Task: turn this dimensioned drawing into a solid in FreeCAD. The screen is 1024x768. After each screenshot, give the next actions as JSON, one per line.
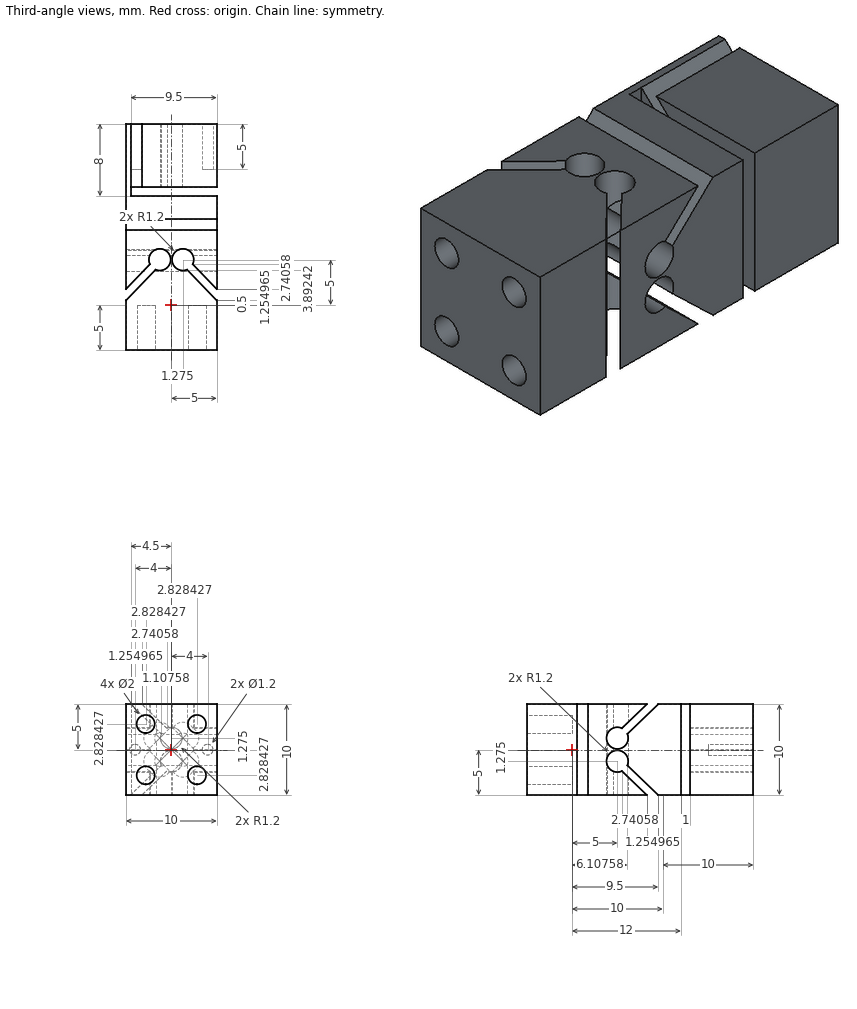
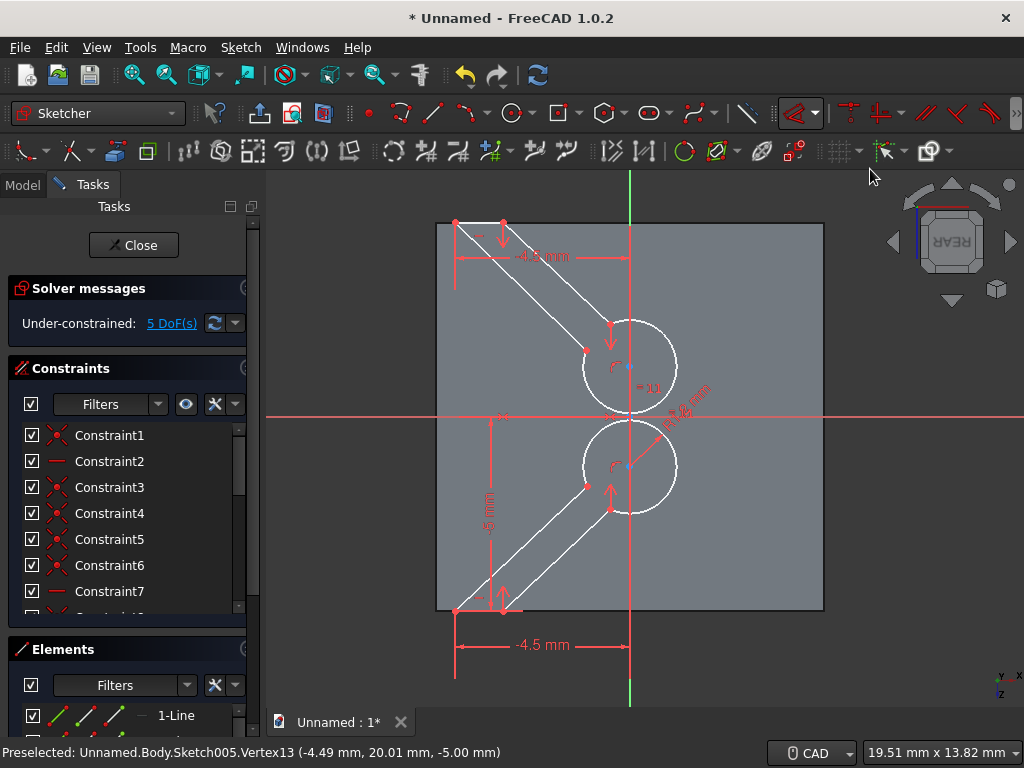
{"action": "left_click", "coordinate": [630, 467]}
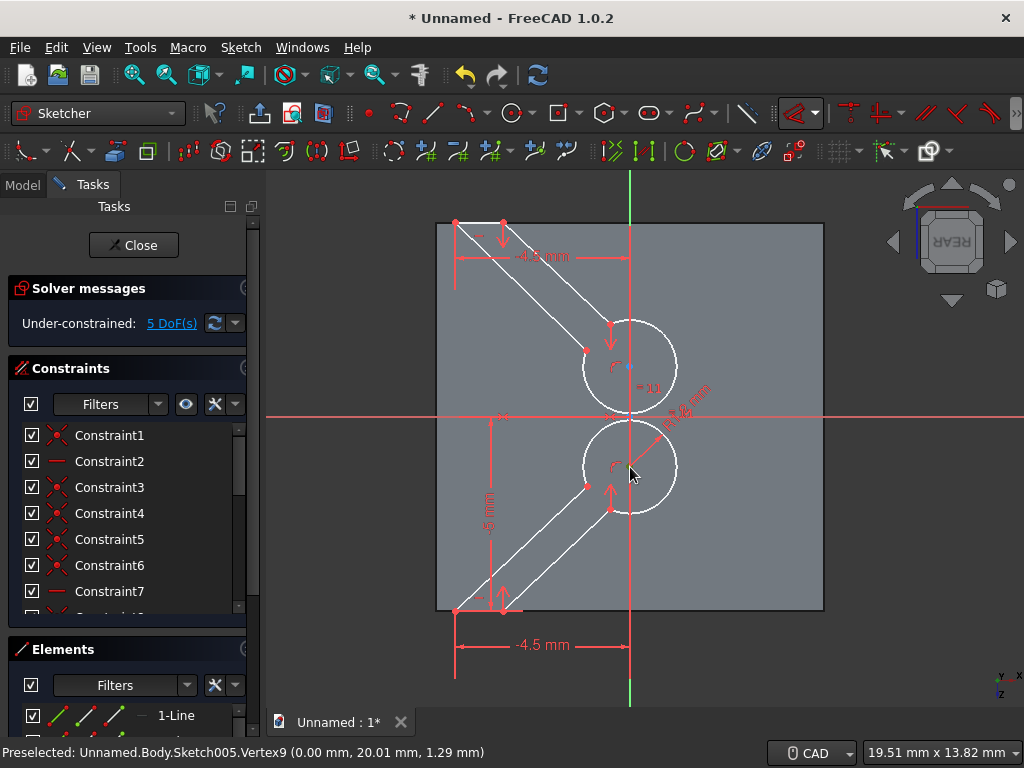
{"action": "key", "text": "i"}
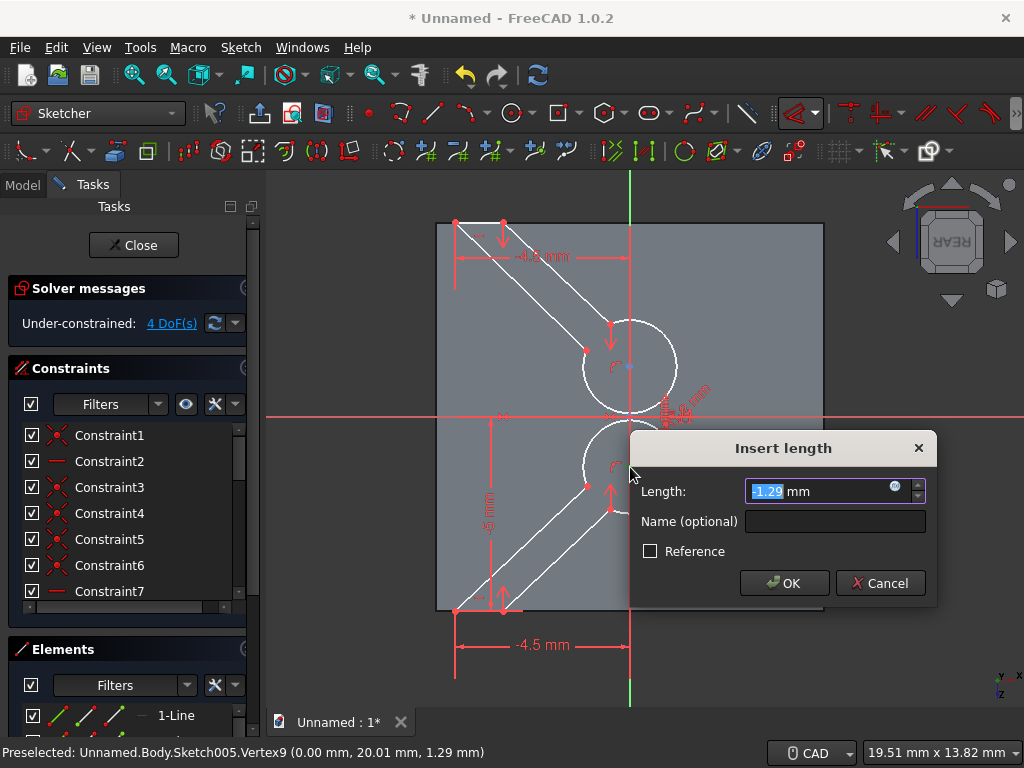
{"action": "type", "text": "-1.275"}
{"action": "key", "text": "Return"}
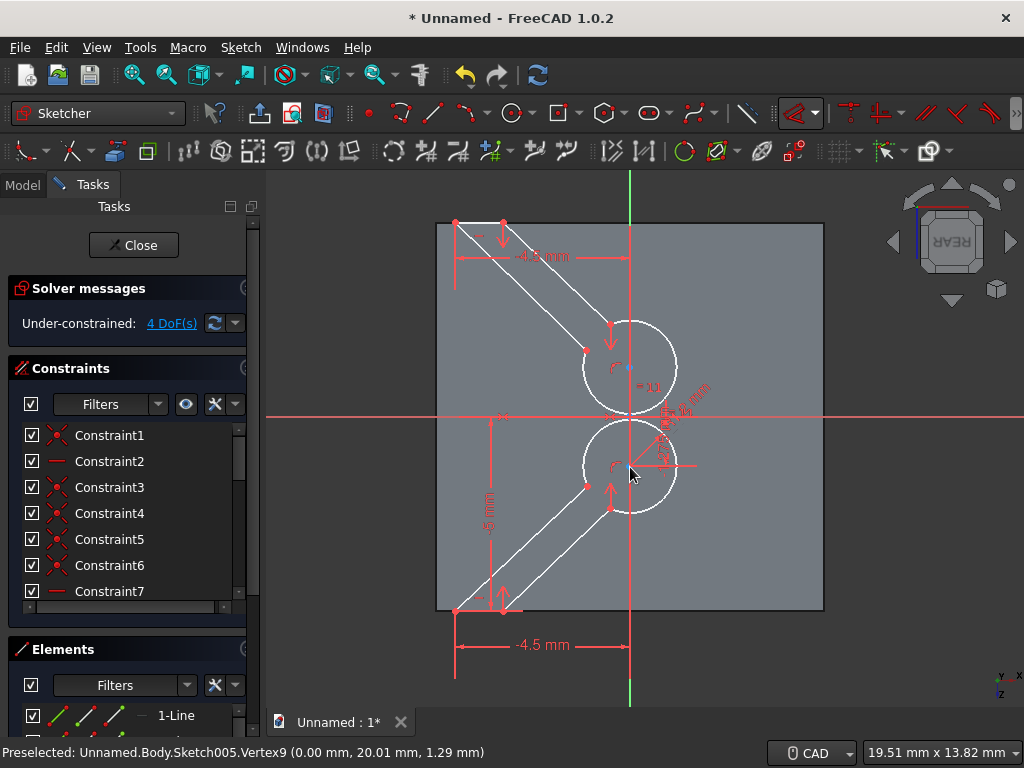
{"action": "scroll", "coordinate": [470, 611], "scroll_direction": "up", "scroll_amount": 2}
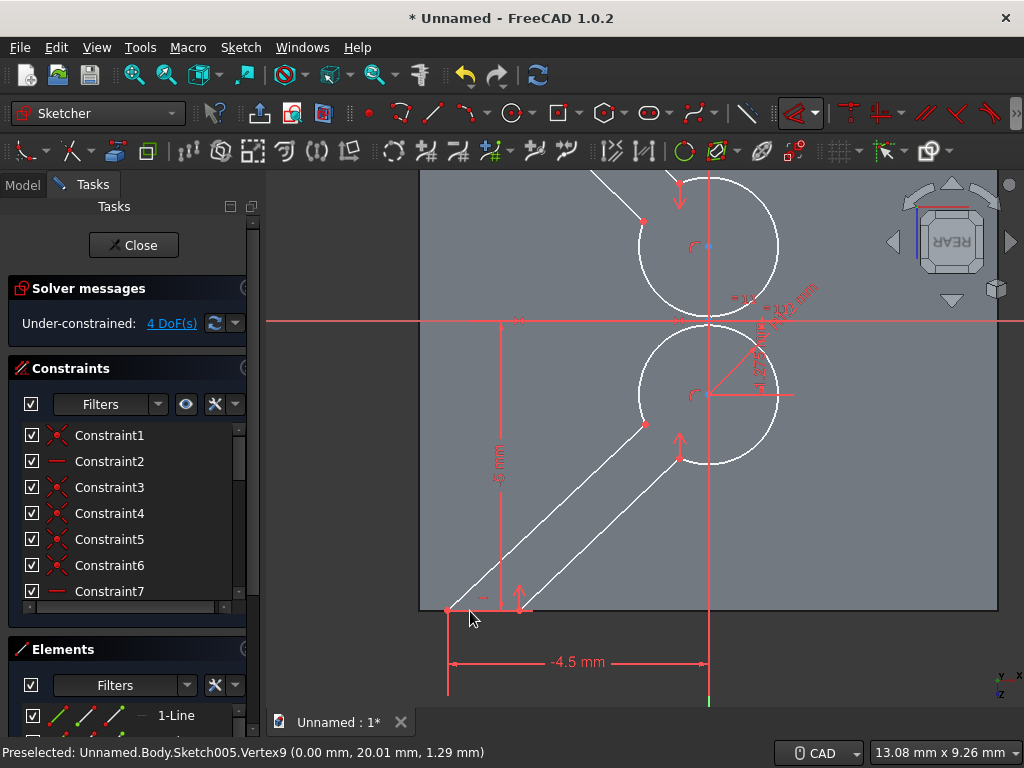
{"action": "left_click", "coordinate": [469, 611]}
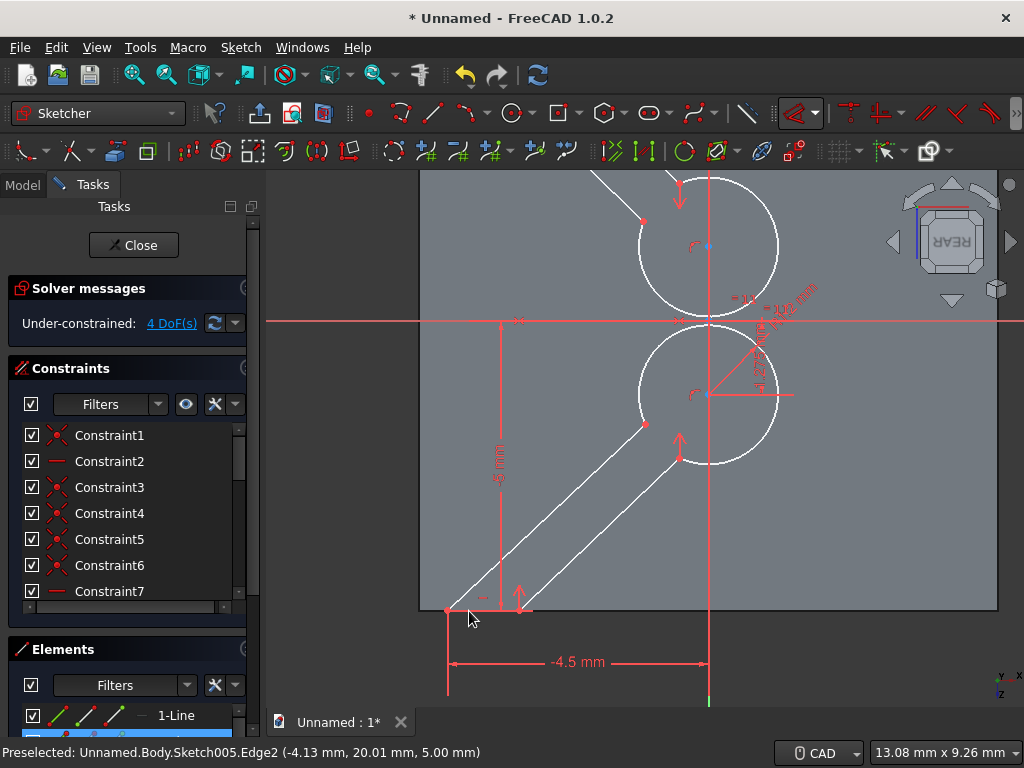
{"action": "key", "text": "l"}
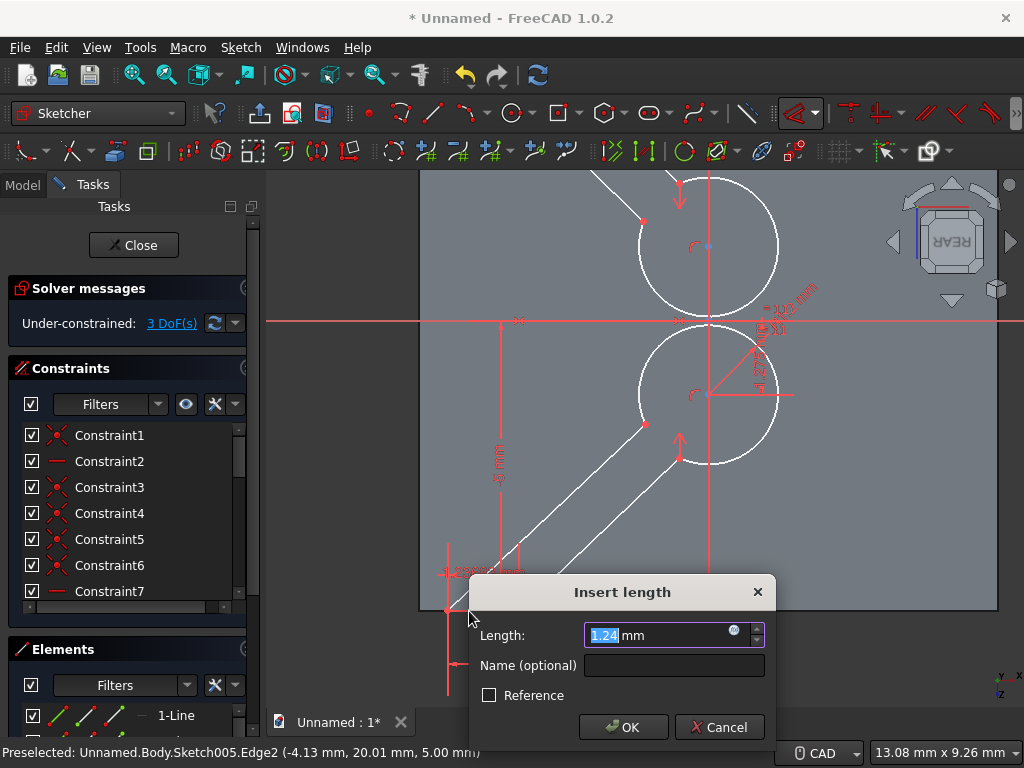
{"action": "type", "text": "1.254965"}
{"action": "key", "text": "Return"}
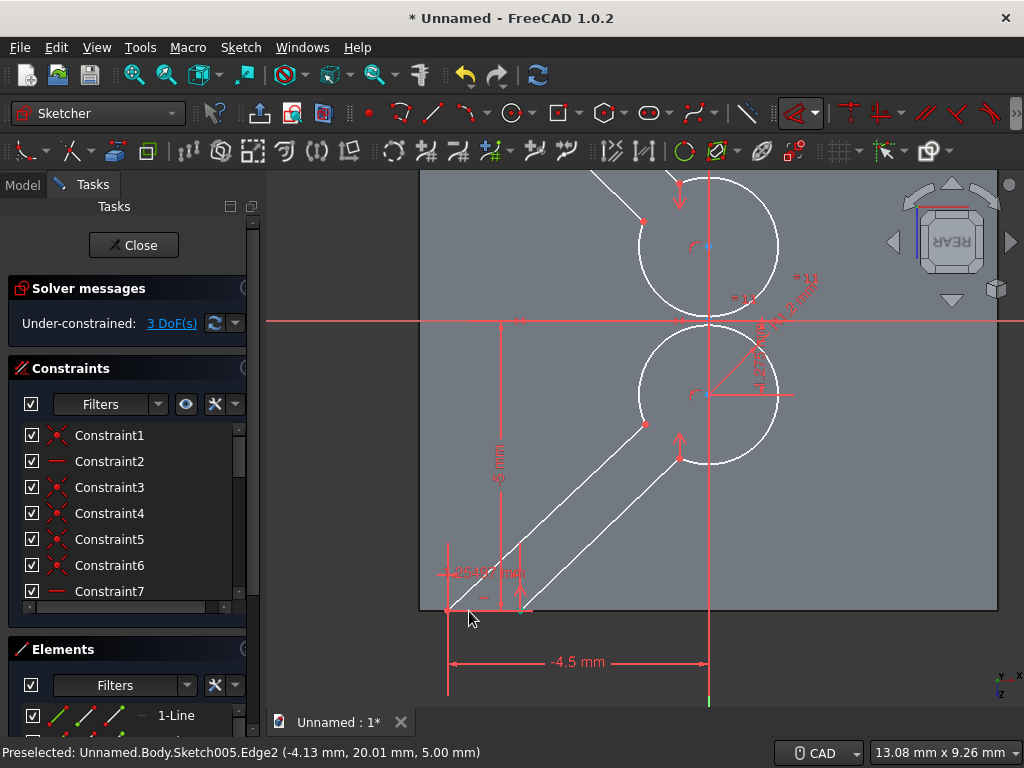
{"action": "left_click", "coordinate": [646, 424]}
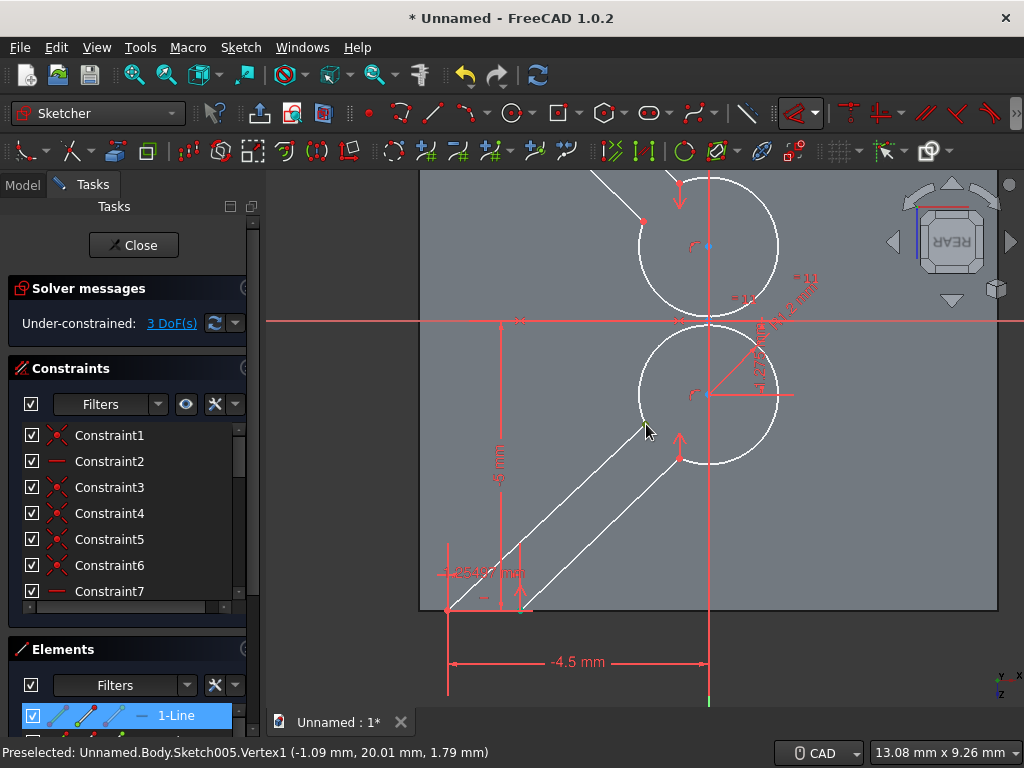
{"action": "key", "text": "l"}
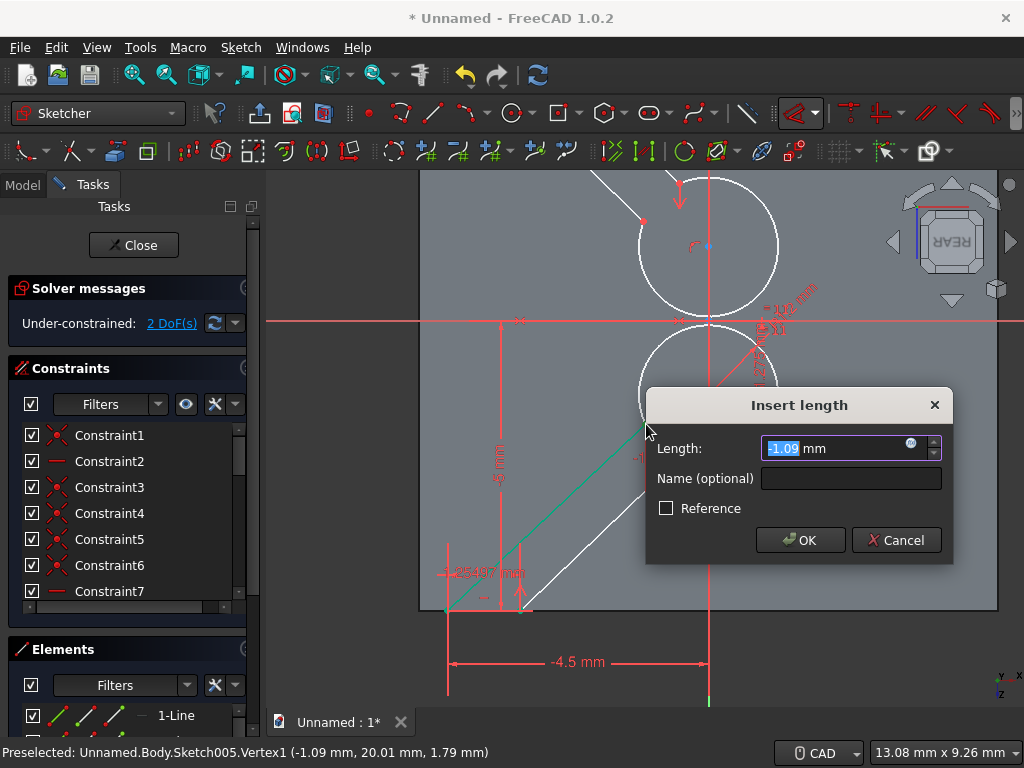
{"action": "type", "text": "-1.10758"}
{"action": "key", "text": "Return"}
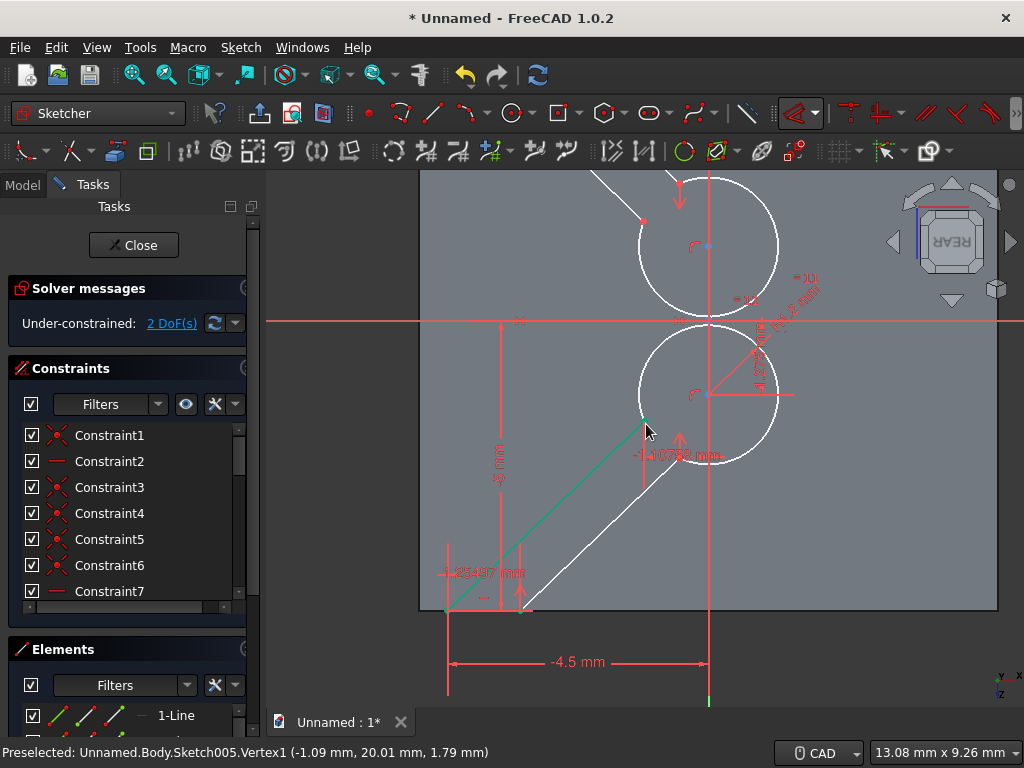
{"action": "left_click", "coordinate": [644, 222]}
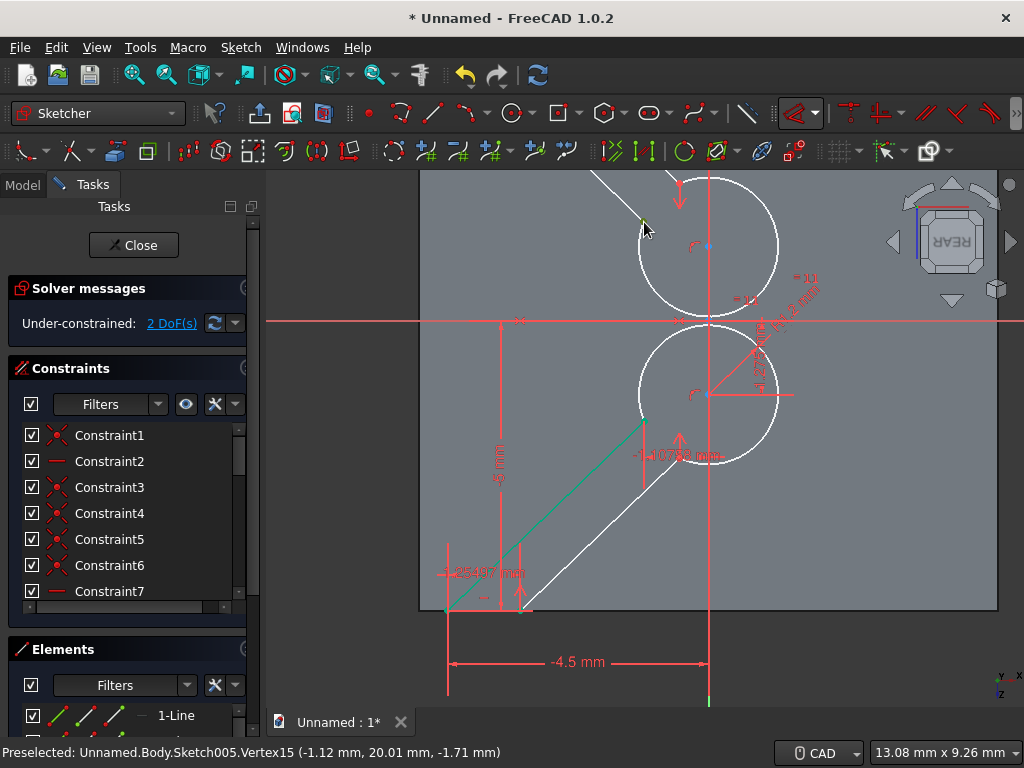
{"action": "left_click", "coordinate": [818, 114]}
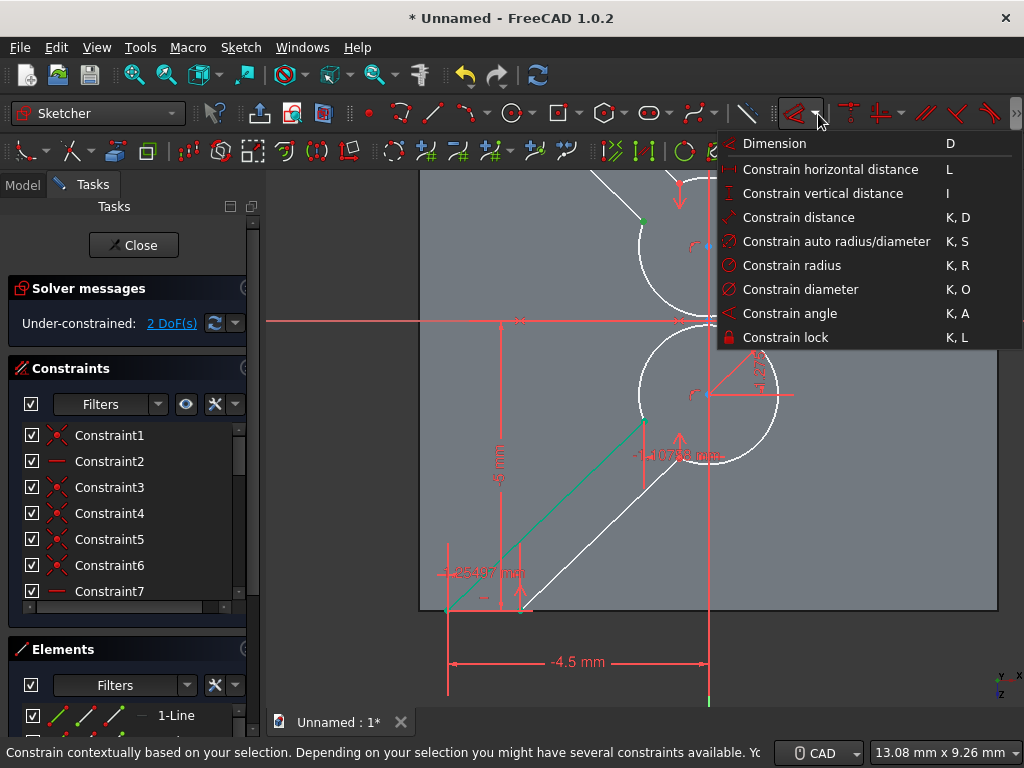
{"action": "left_click", "coordinate": [870, 169]}